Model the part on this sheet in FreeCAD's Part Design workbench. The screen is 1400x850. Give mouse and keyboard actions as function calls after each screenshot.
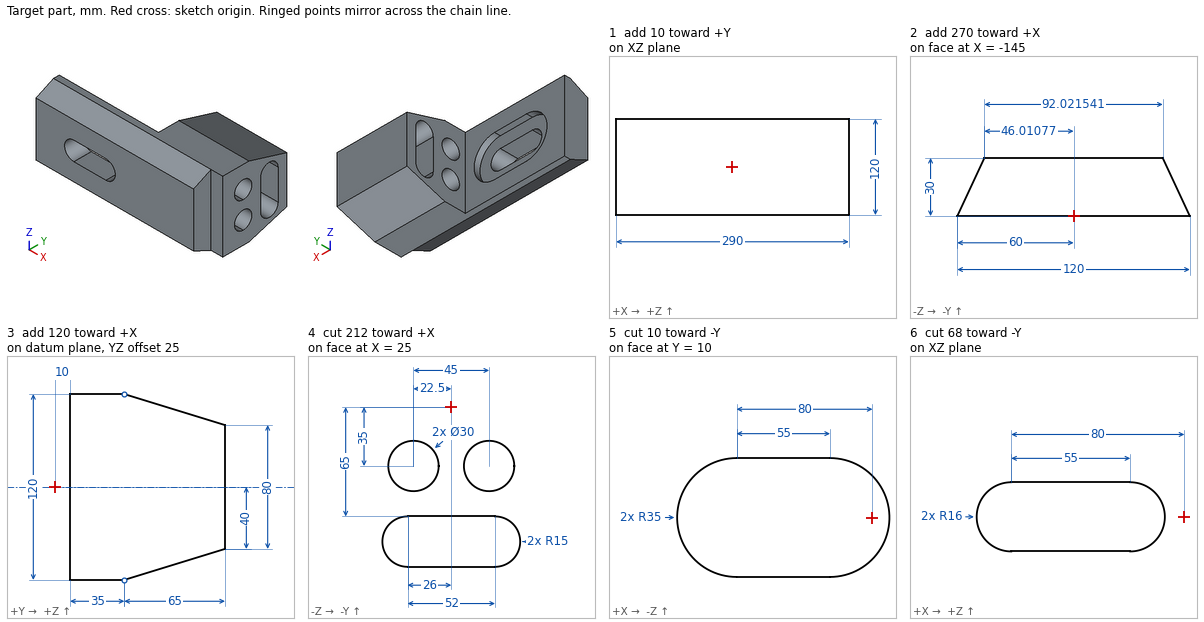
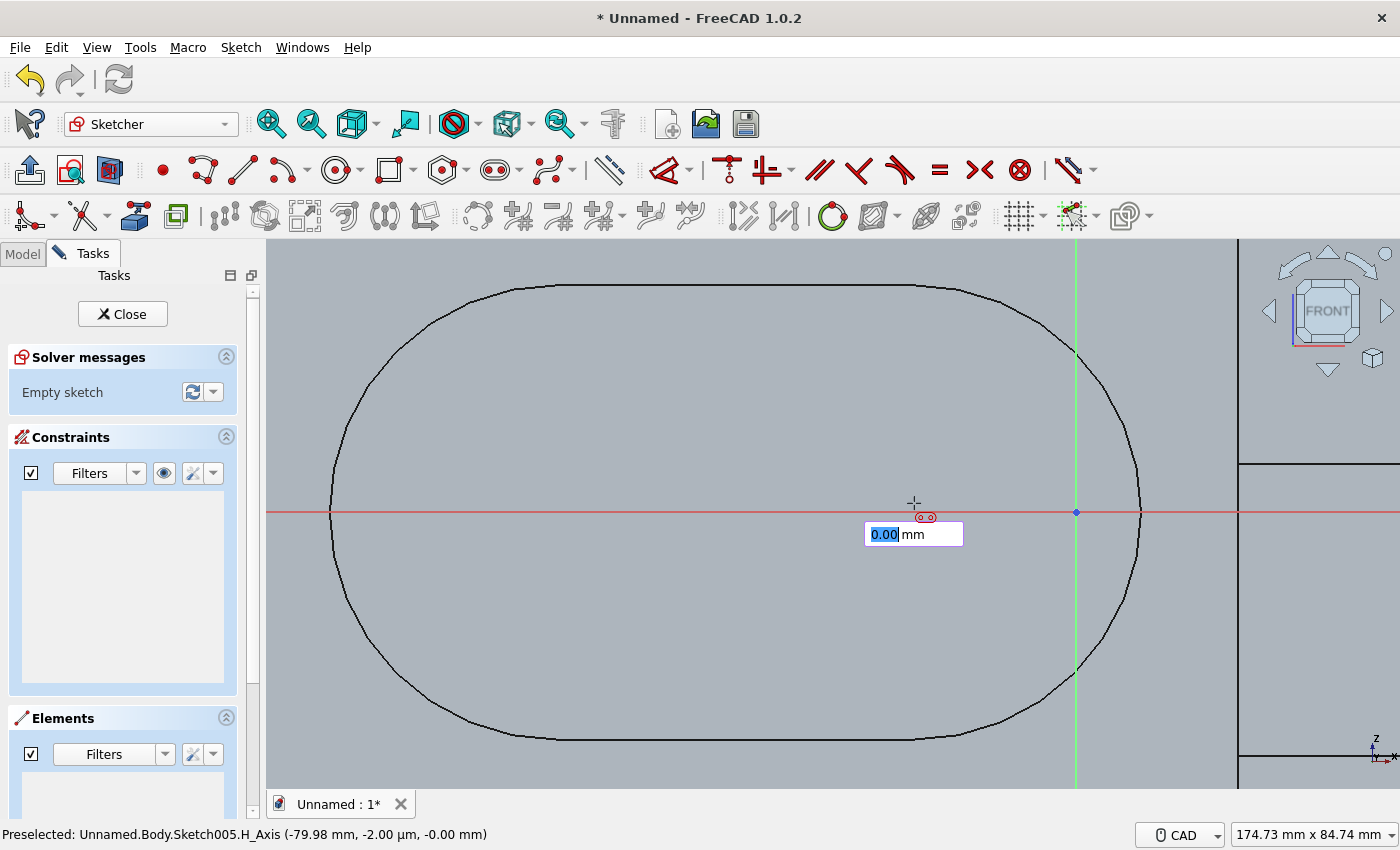
click(735, 616)
key(Escape)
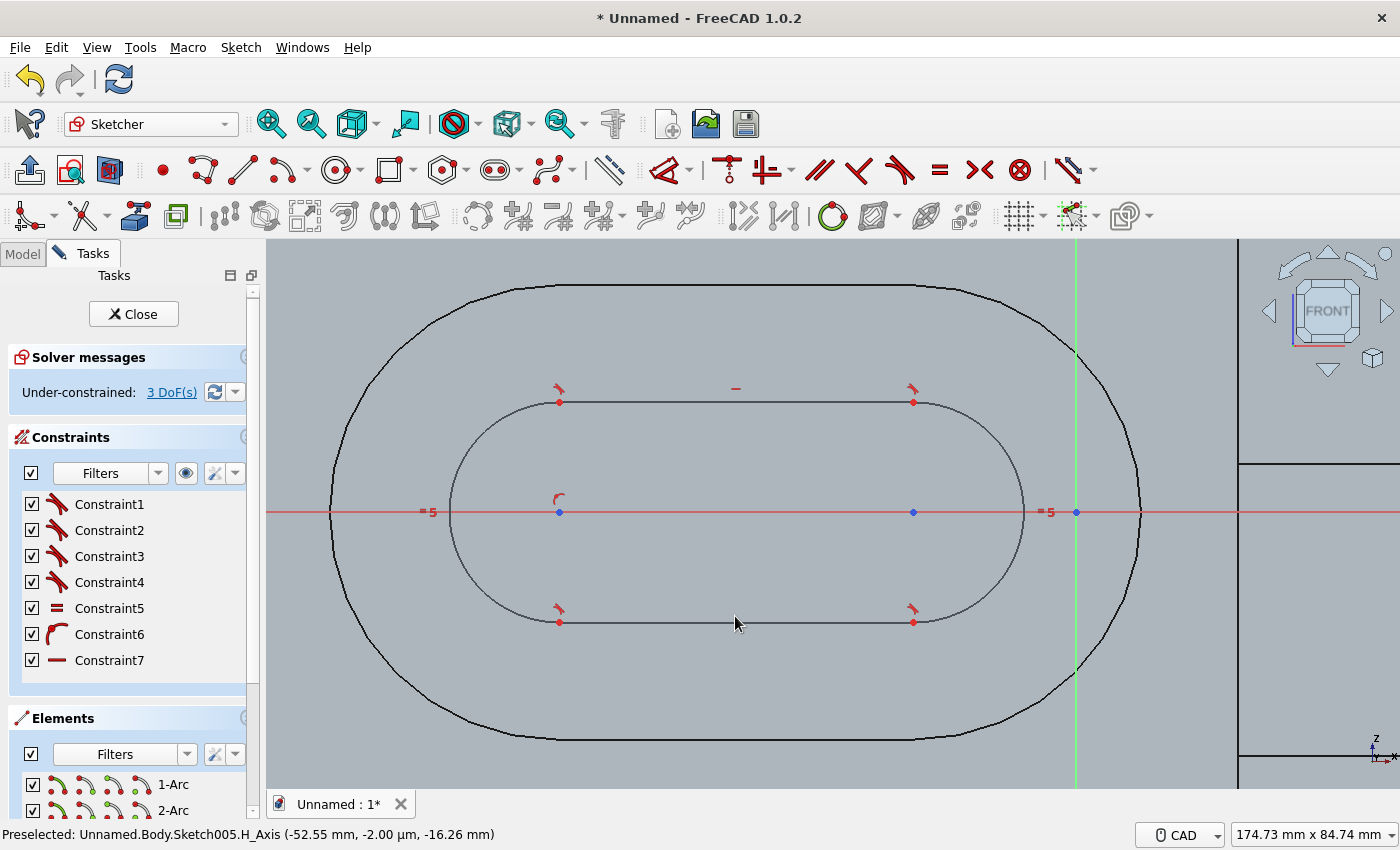
key(d)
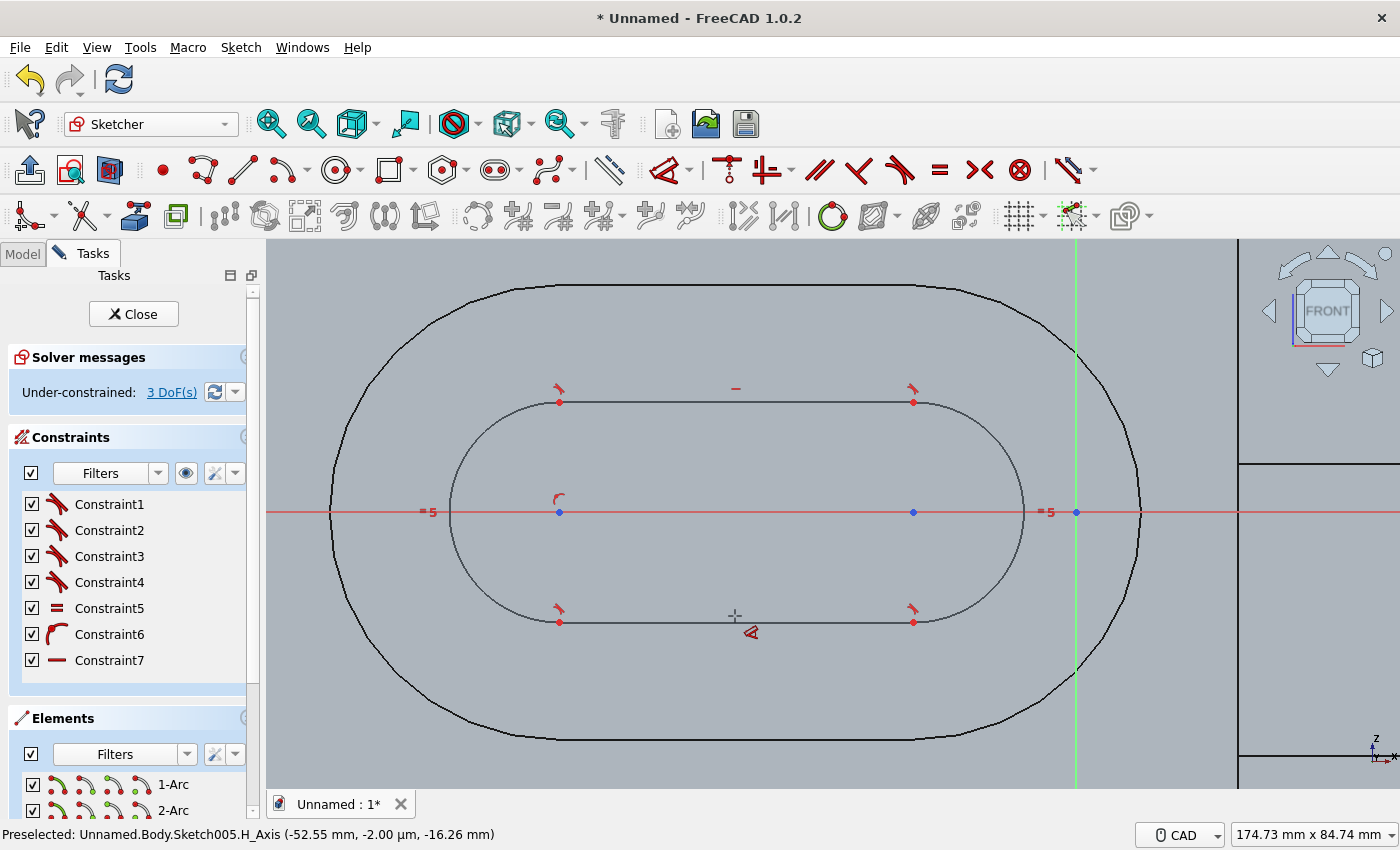
click(471, 448)
click(445, 429)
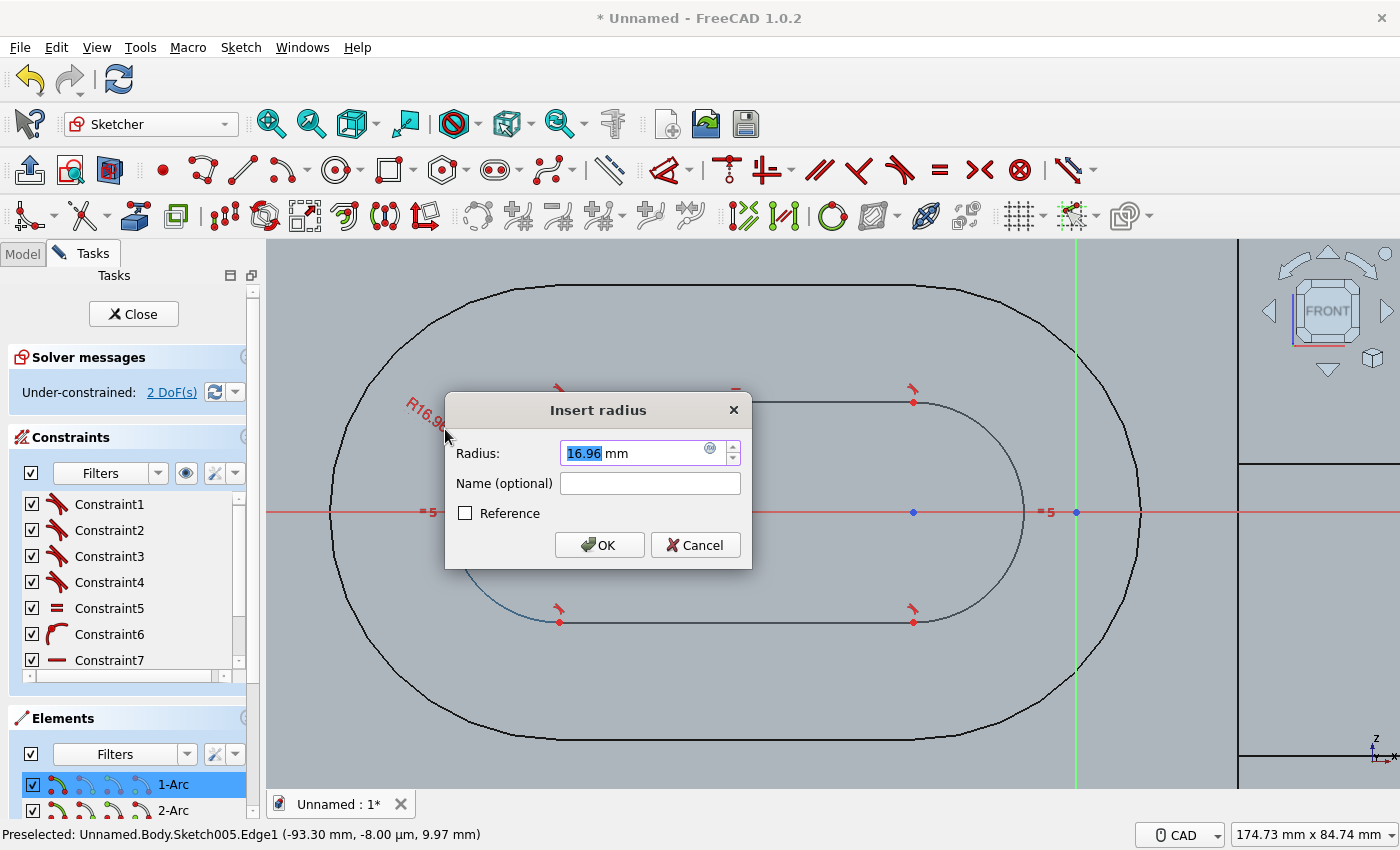
text(16)
key(Return)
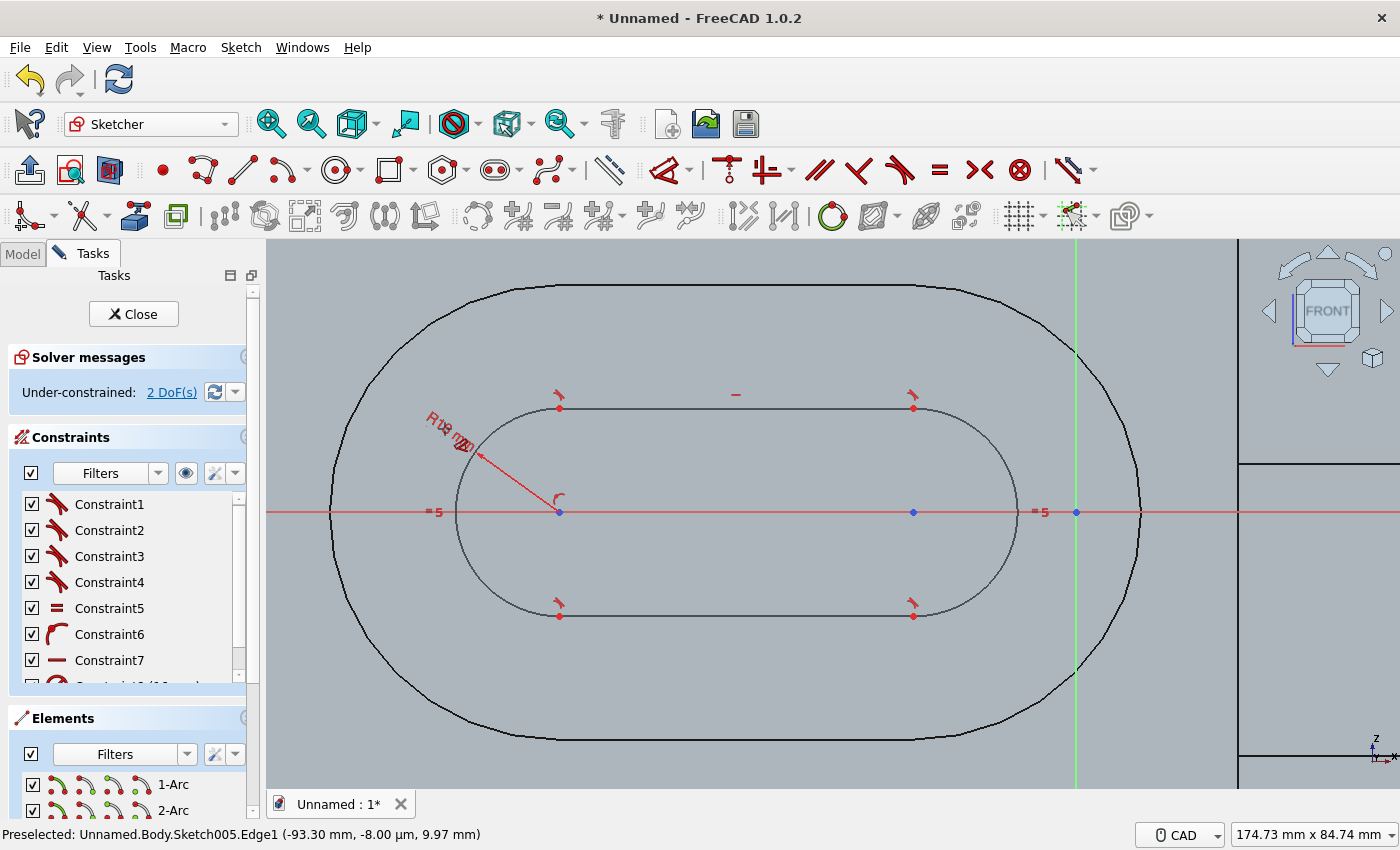
click(666, 409)
click(737, 375)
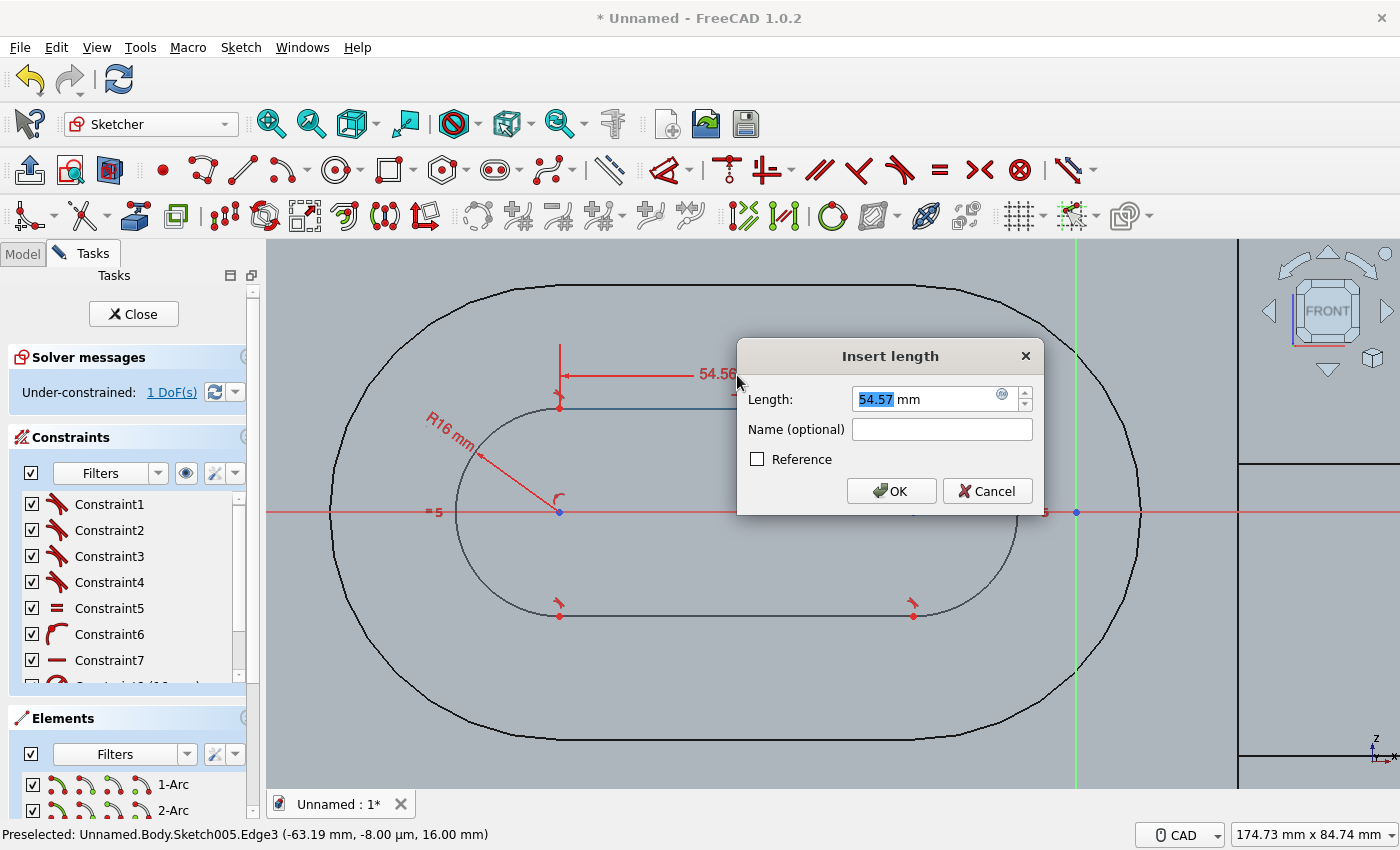
text(55)
key(Return)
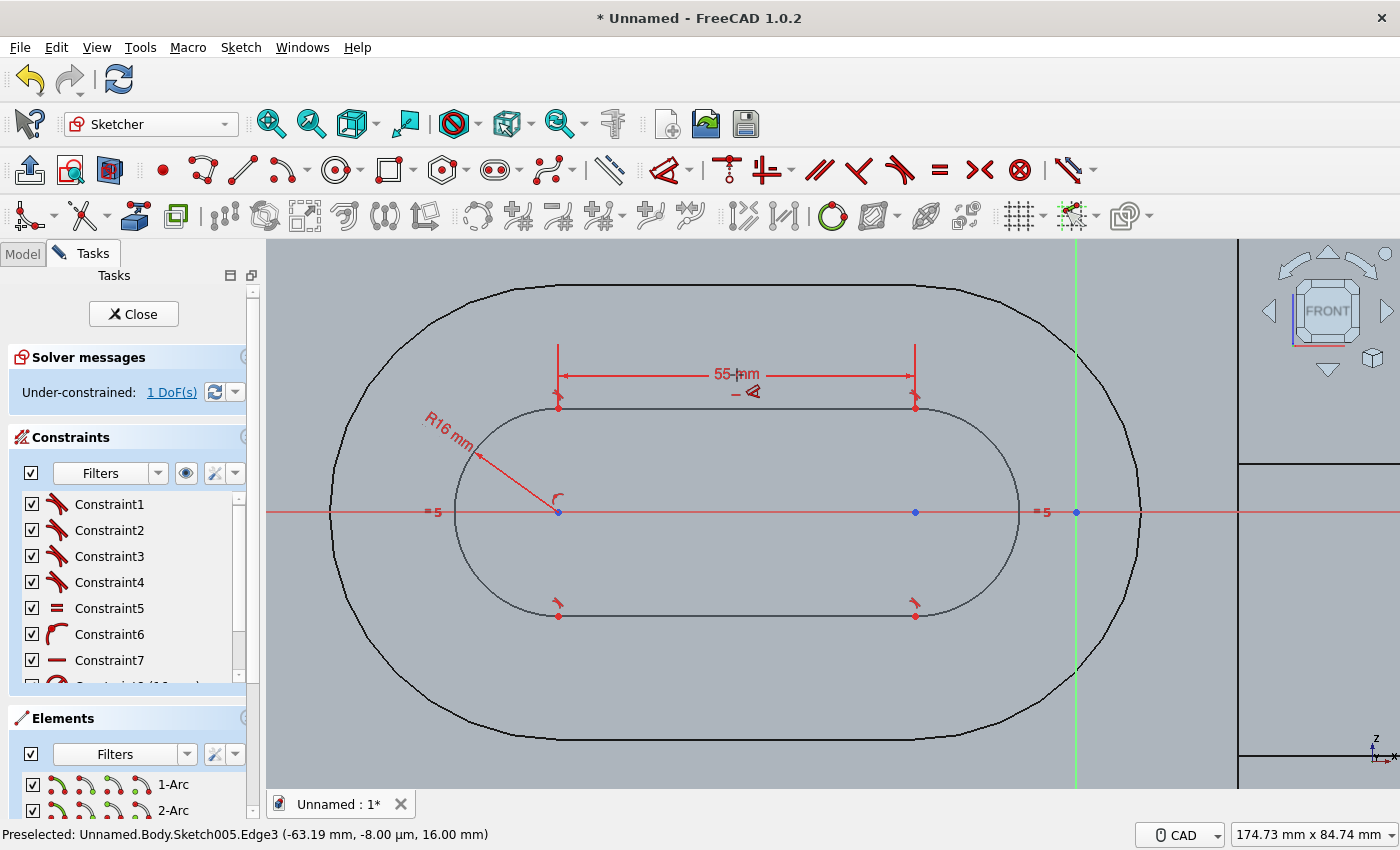
click(558, 409)
click(817, 375)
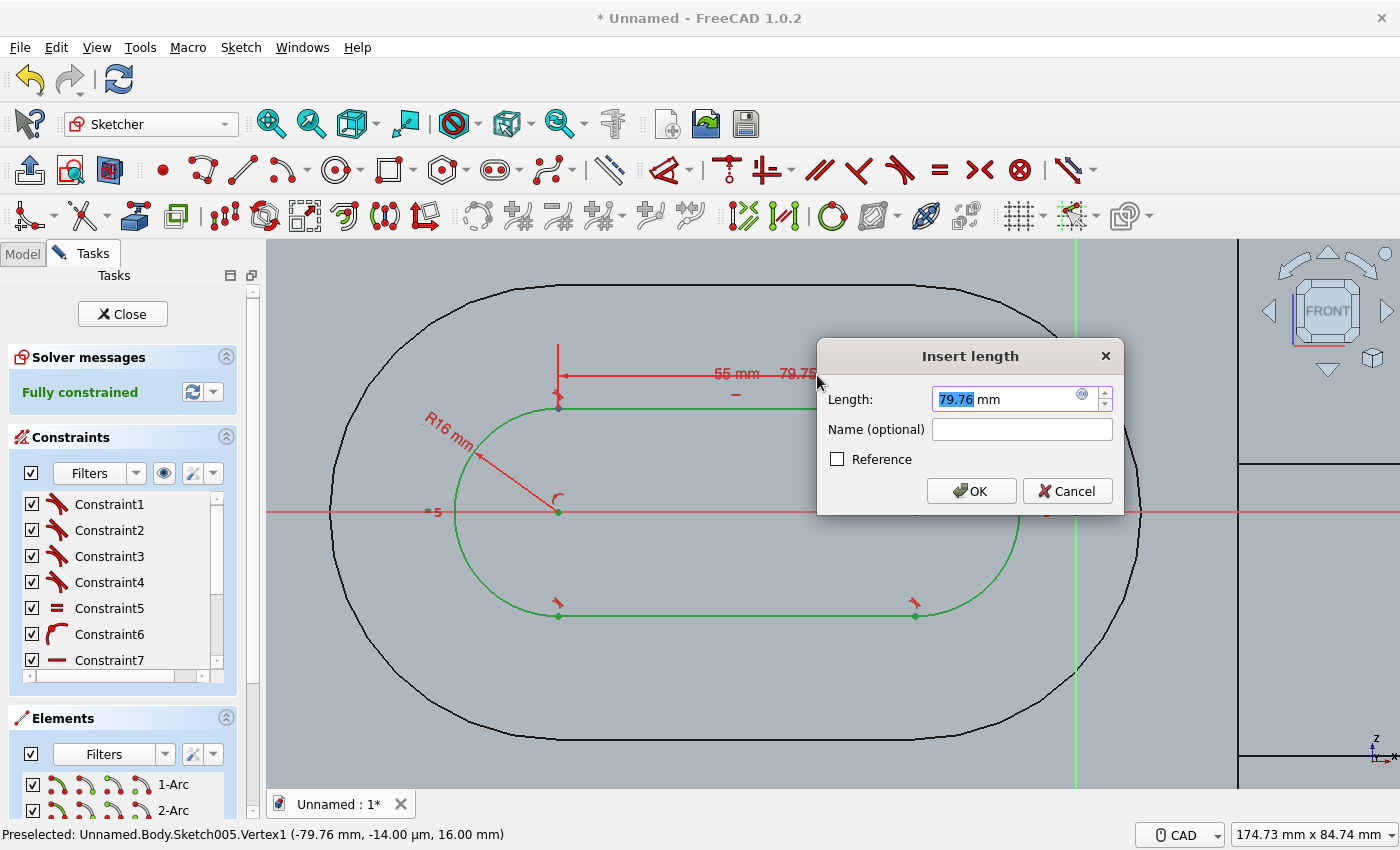
text(80)
key(Return)
key(Escape)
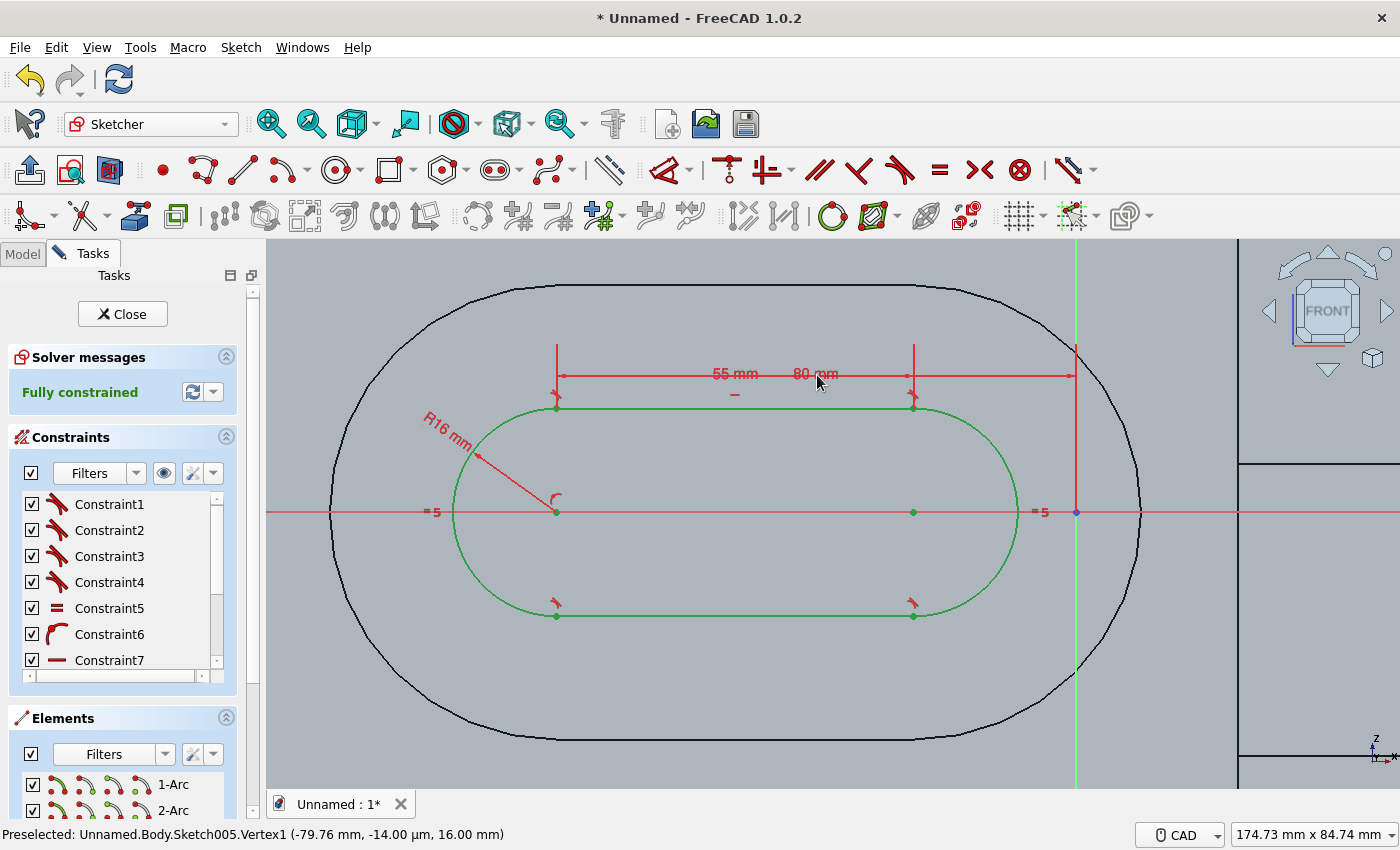
click(123, 314)